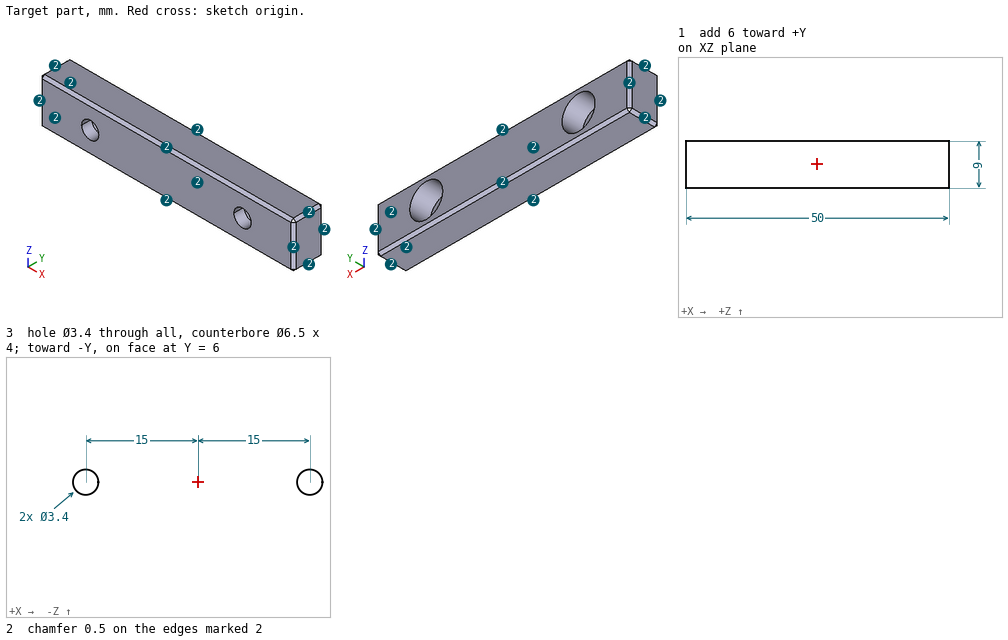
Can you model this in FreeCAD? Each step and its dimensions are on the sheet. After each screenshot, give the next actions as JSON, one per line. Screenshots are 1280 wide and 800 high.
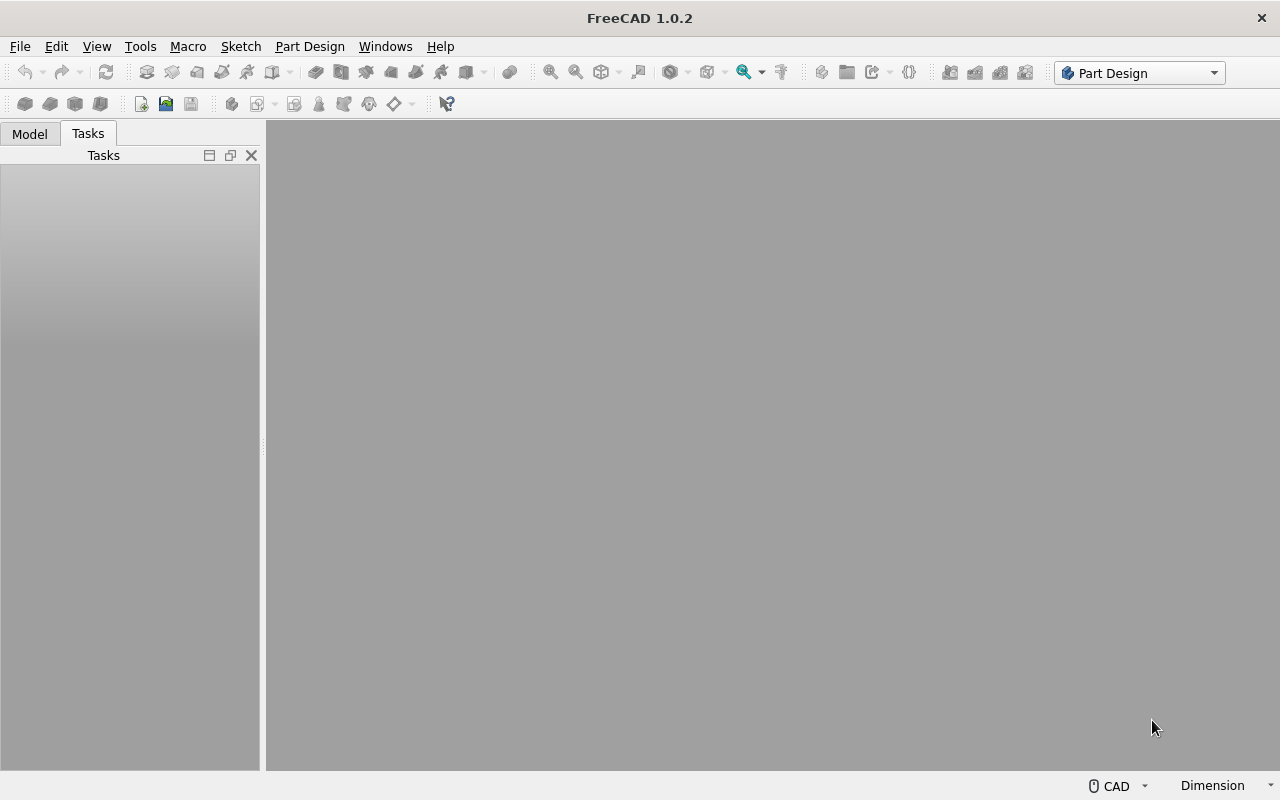
{"action": "left_click", "coordinate": [141, 104]}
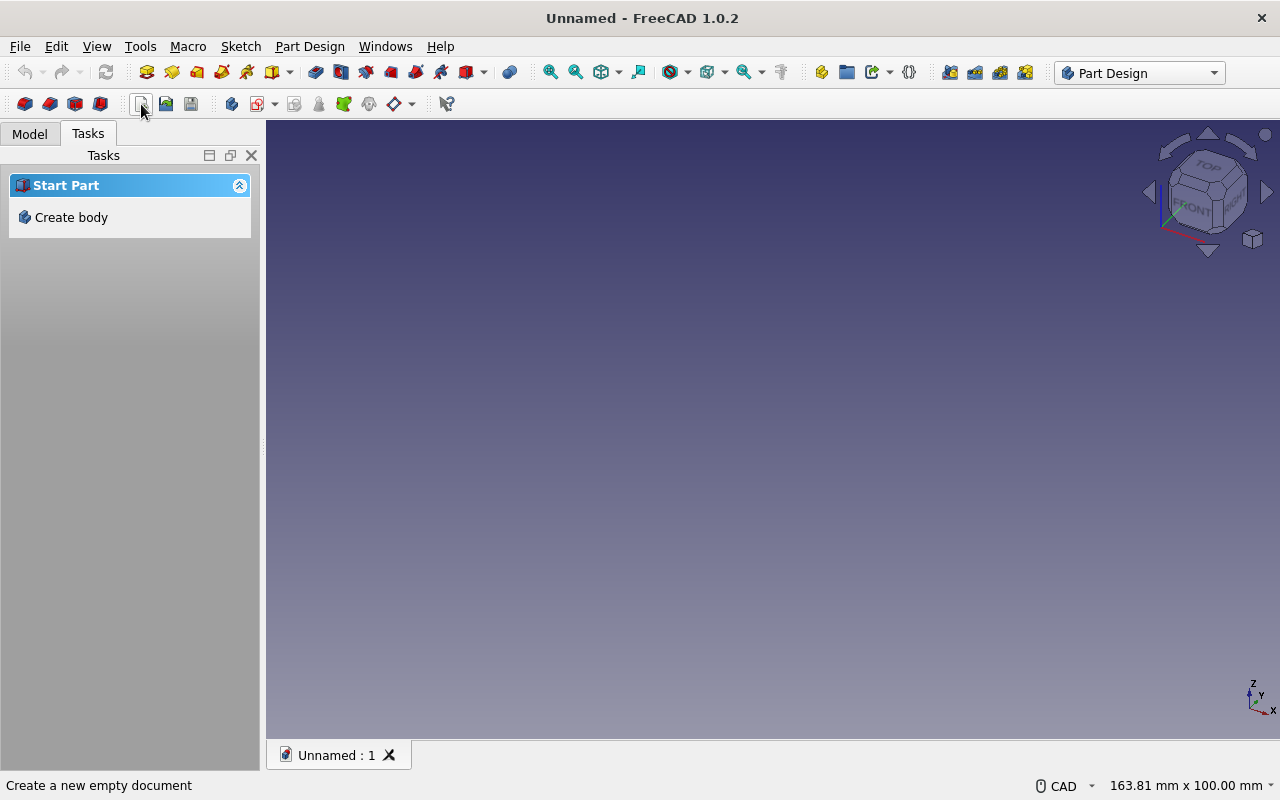
{"action": "left_click", "coordinate": [256, 104]}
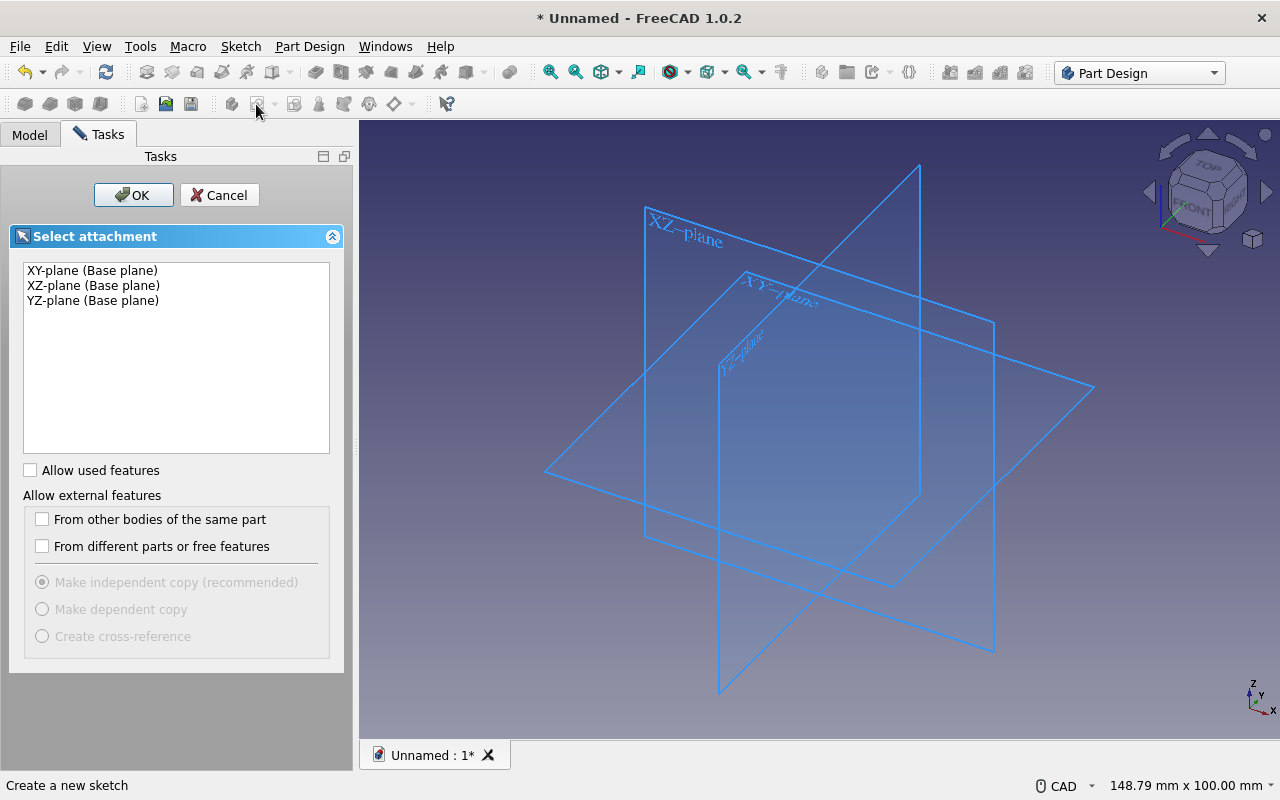
{"action": "left_click", "coordinate": [84, 286]}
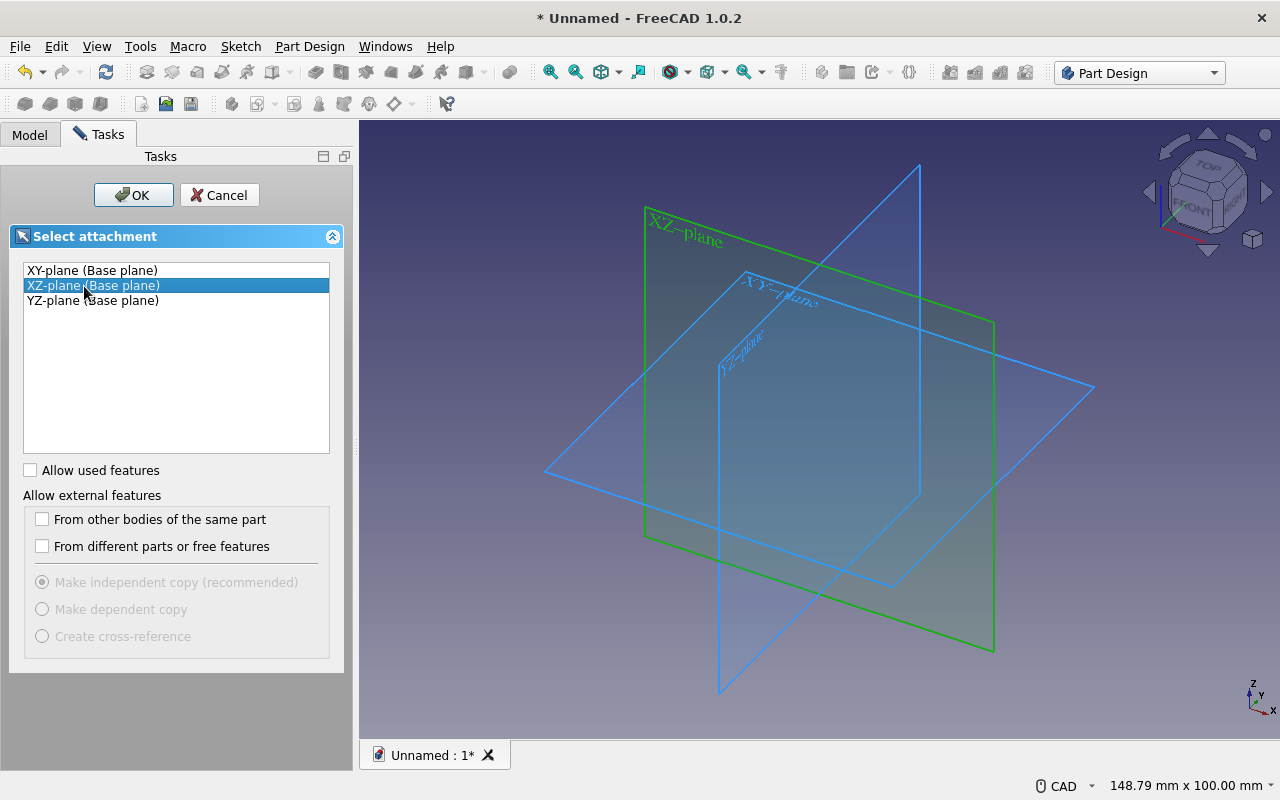
{"action": "left_click", "coordinate": [134, 195]}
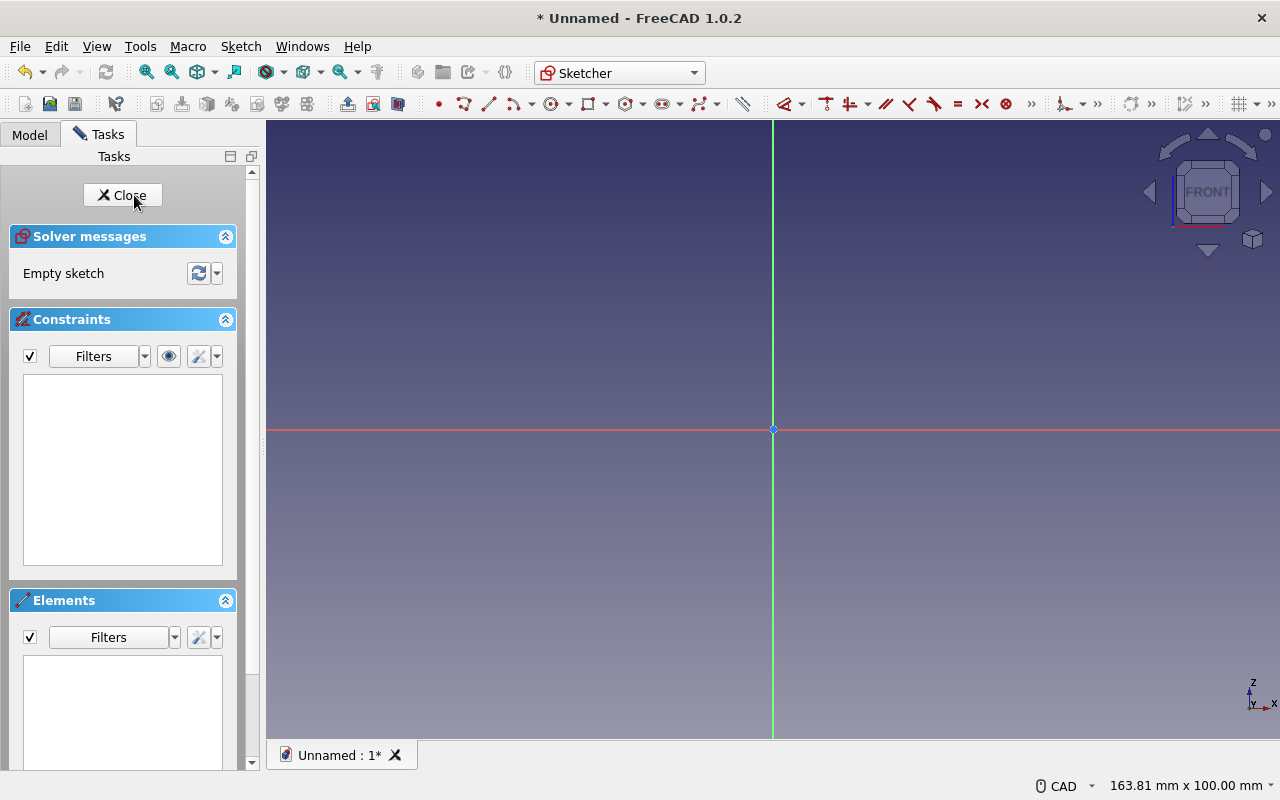
{"action": "scroll", "coordinate": [856, 430], "scroll_direction": "up", "scroll_amount": 3}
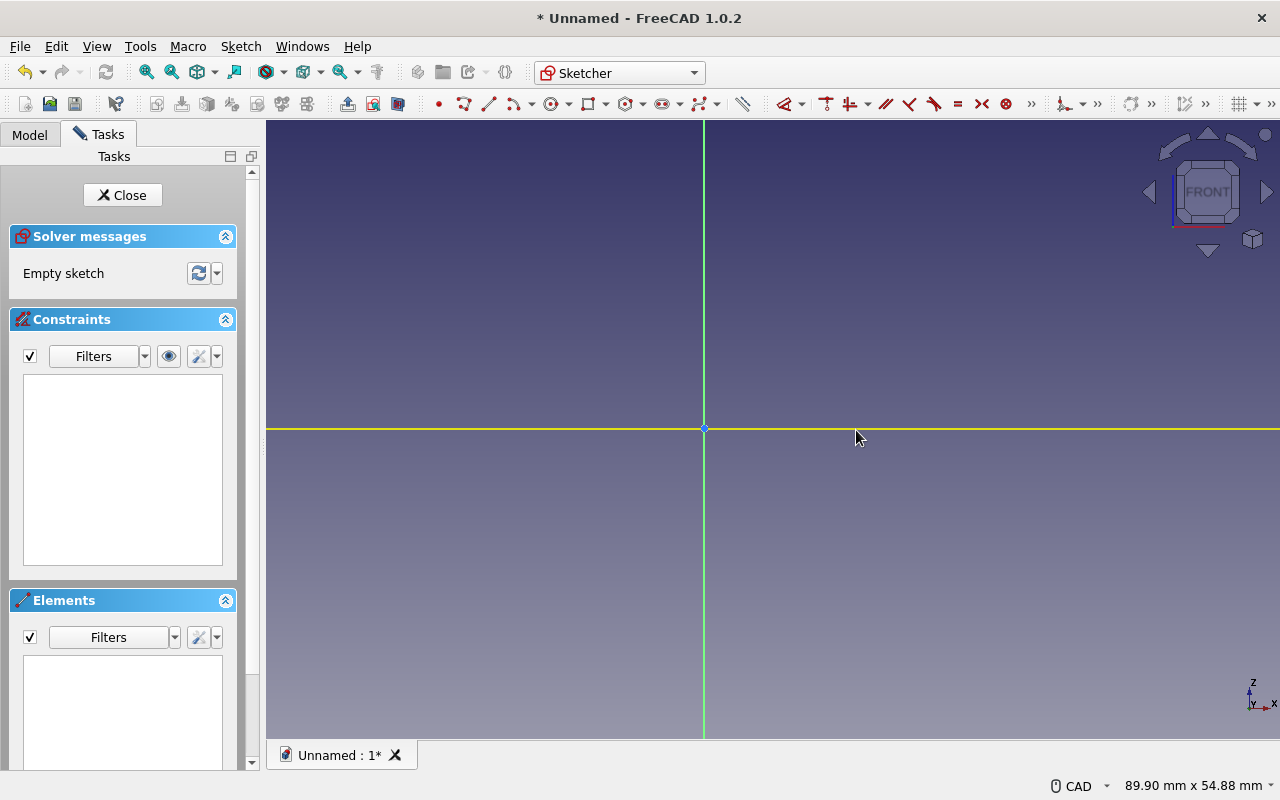
{"action": "left_click", "coordinate": [606, 104]}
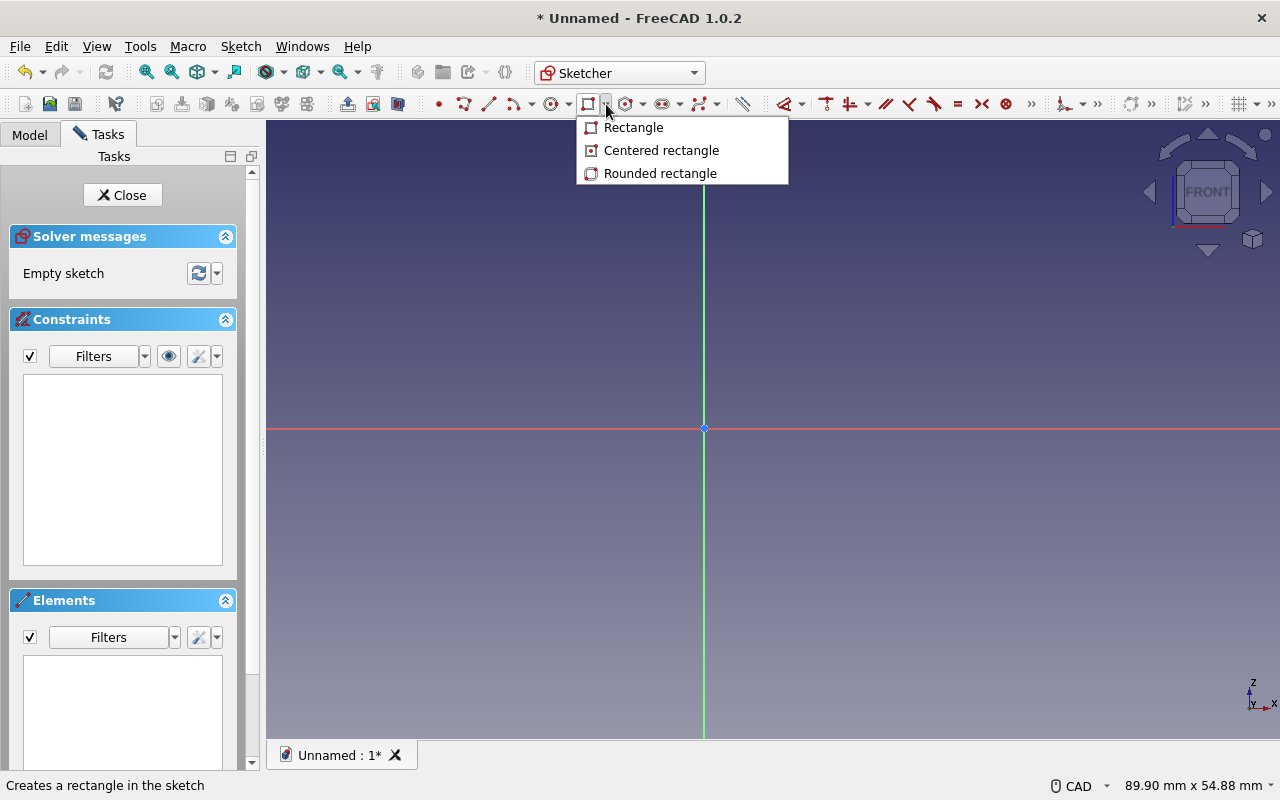
{"action": "left_click", "coordinate": [682, 150]}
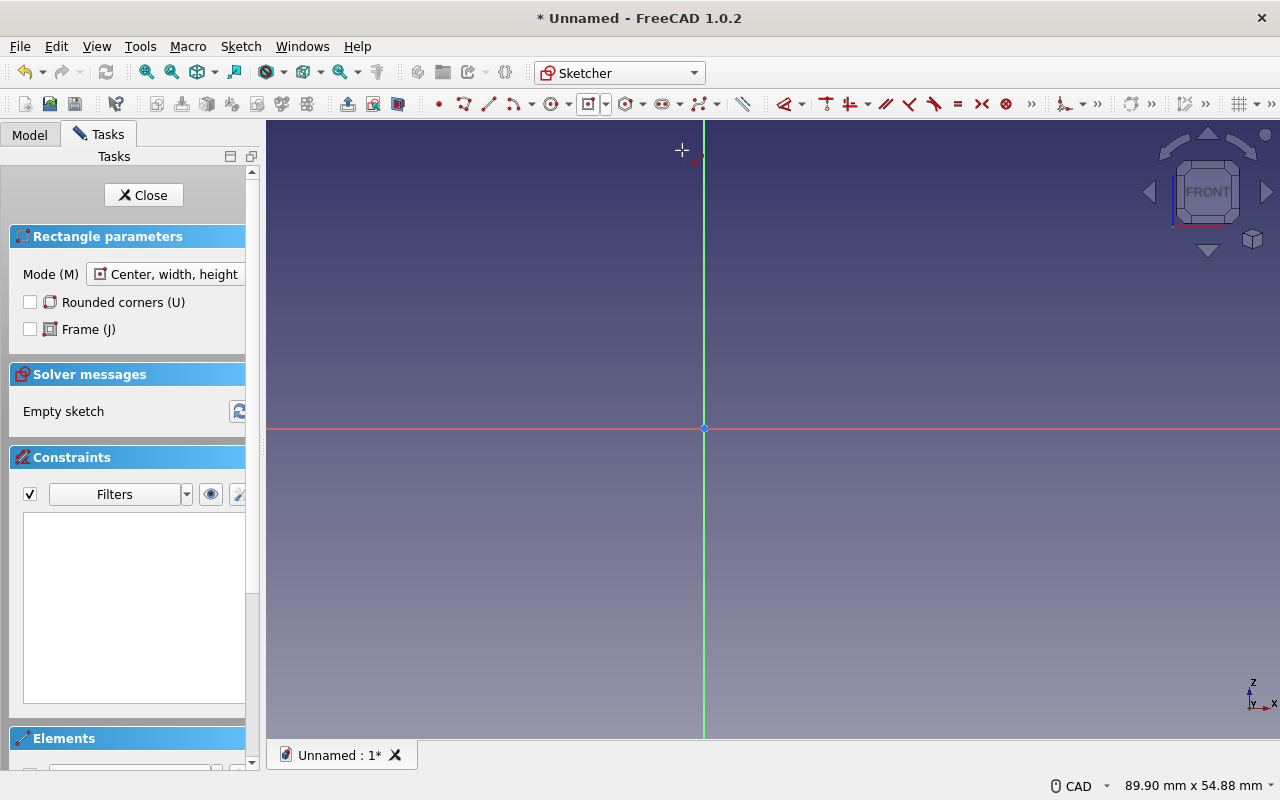
{"action": "left_click", "coordinate": [704, 429]}
{"action": "left_click", "coordinate": [986, 378]}
{"action": "key", "text": "Escape"}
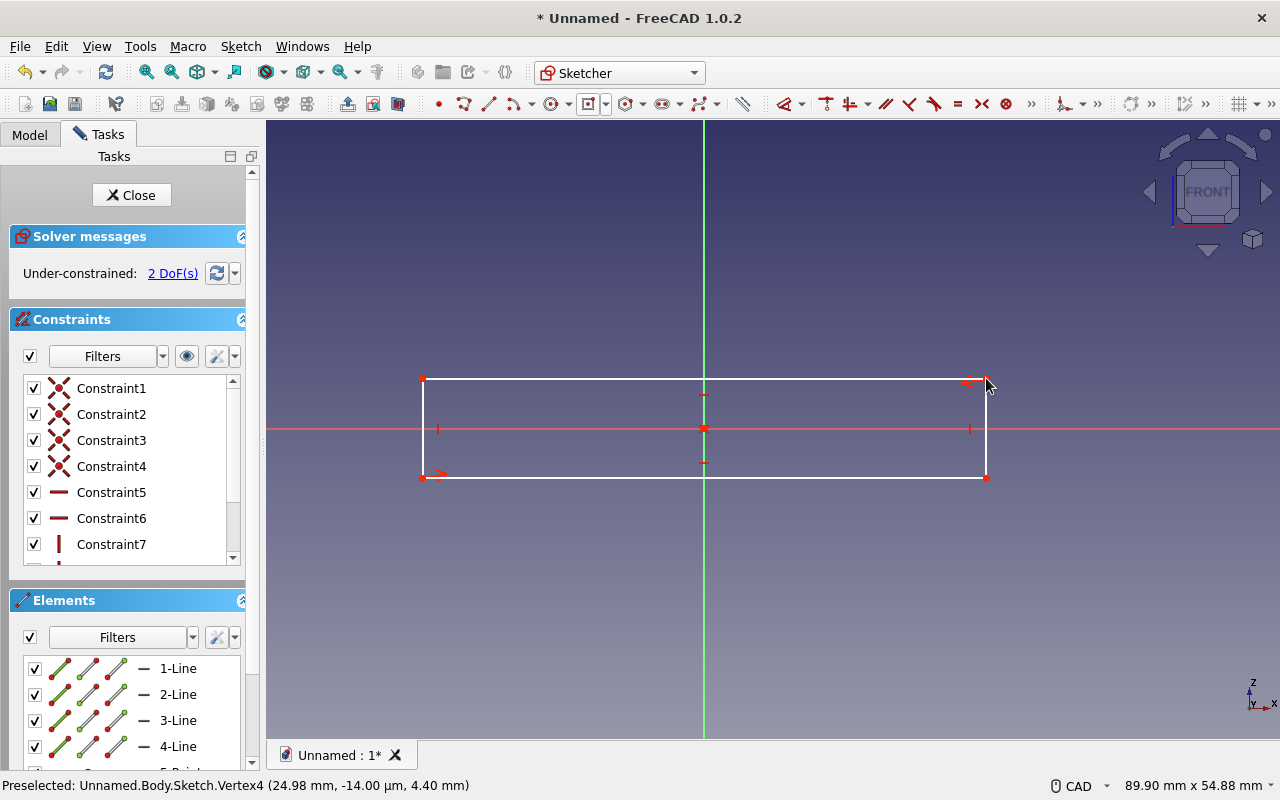
{"action": "left_click", "coordinate": [986, 449]}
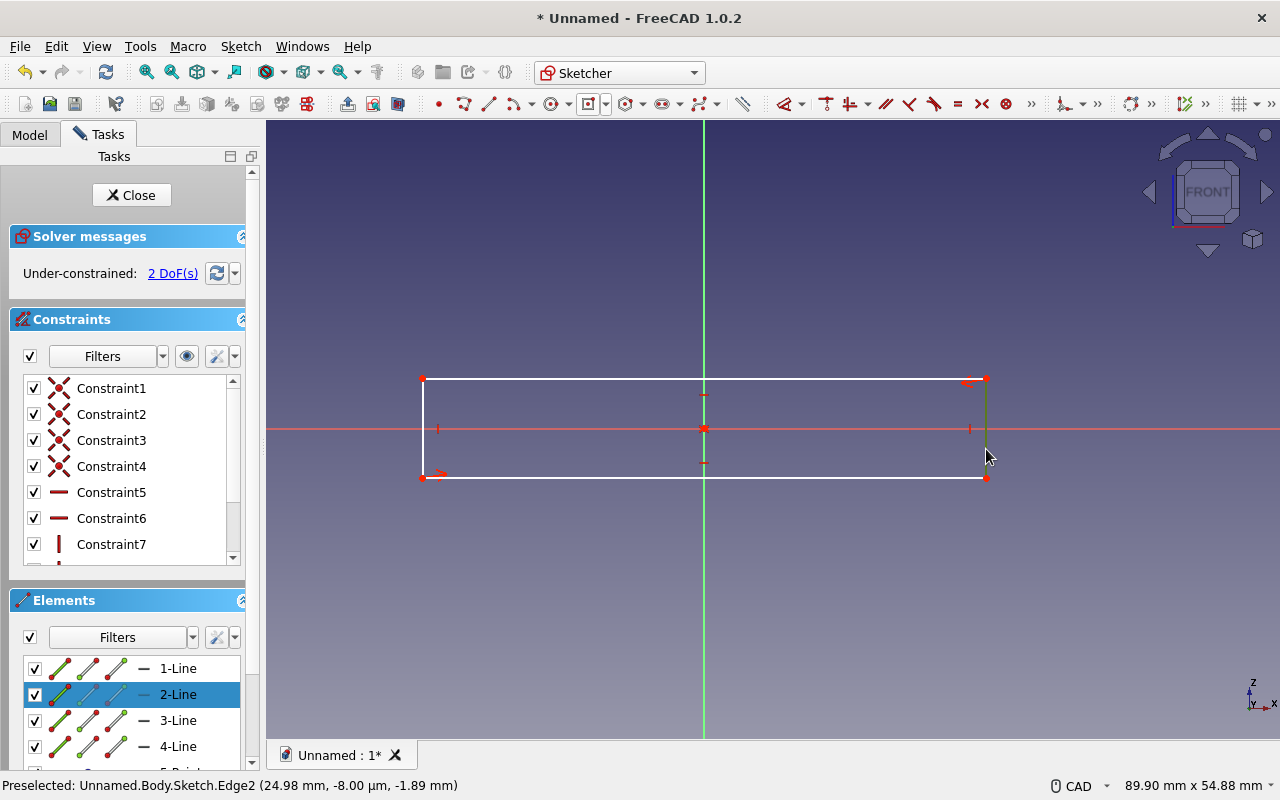
{"action": "key", "text": "i"}